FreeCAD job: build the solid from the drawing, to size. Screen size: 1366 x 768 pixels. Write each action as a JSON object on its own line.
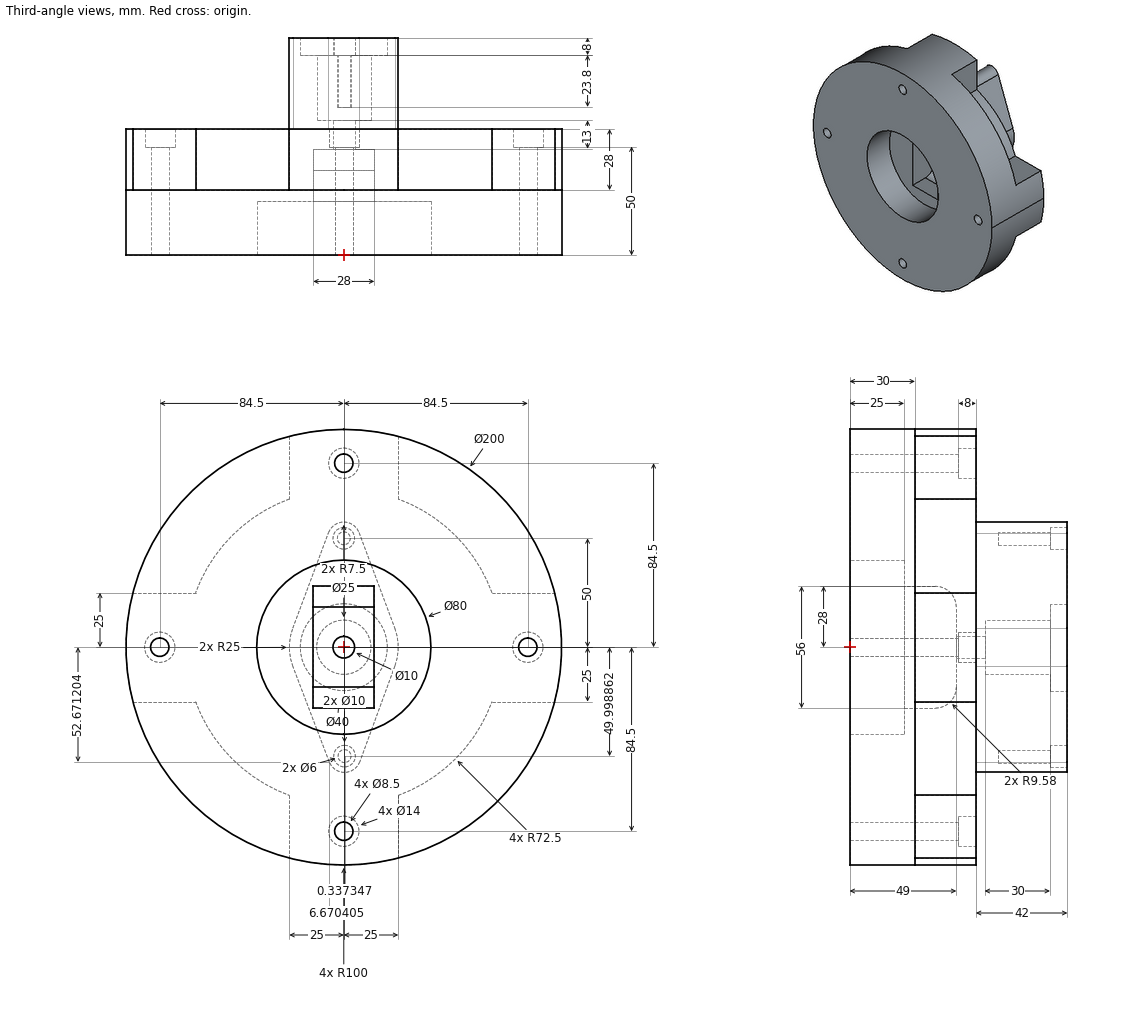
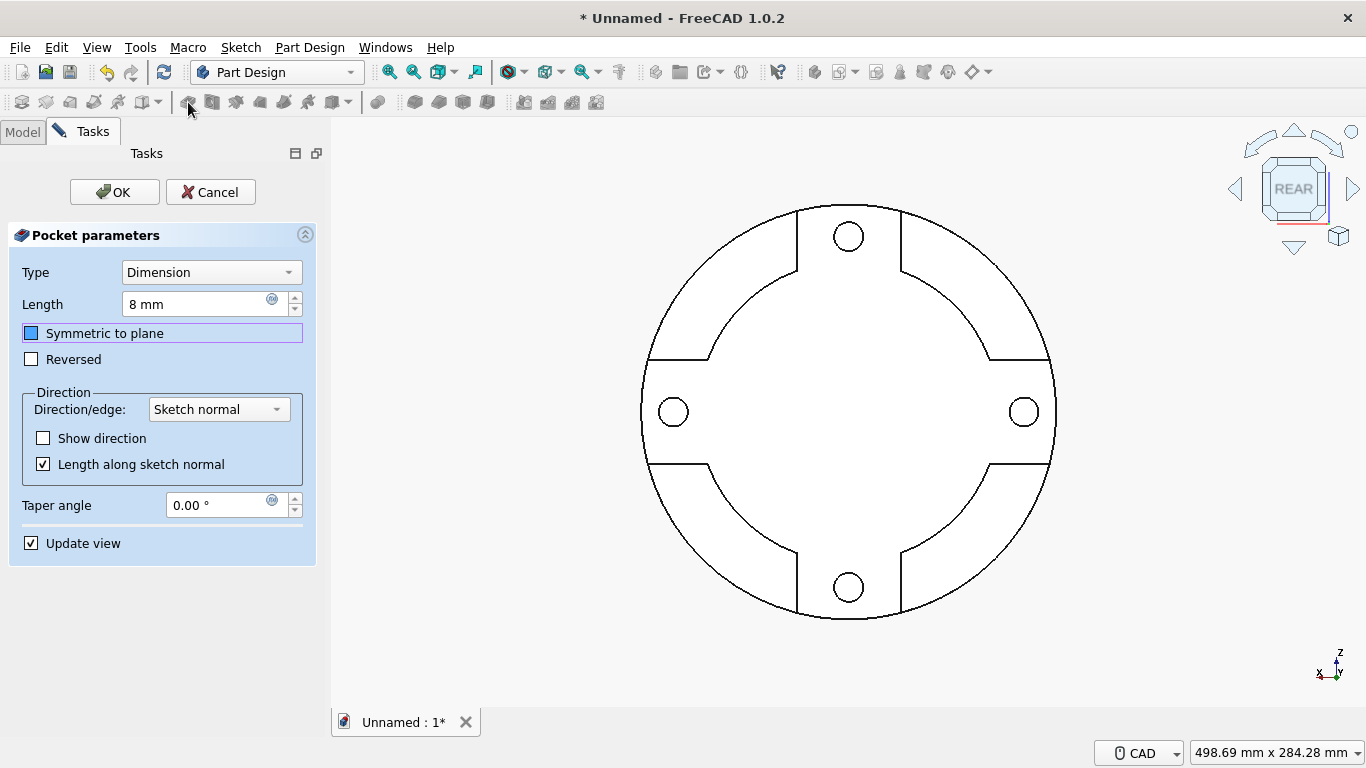
{"action": "left_click", "coordinate": [115, 192]}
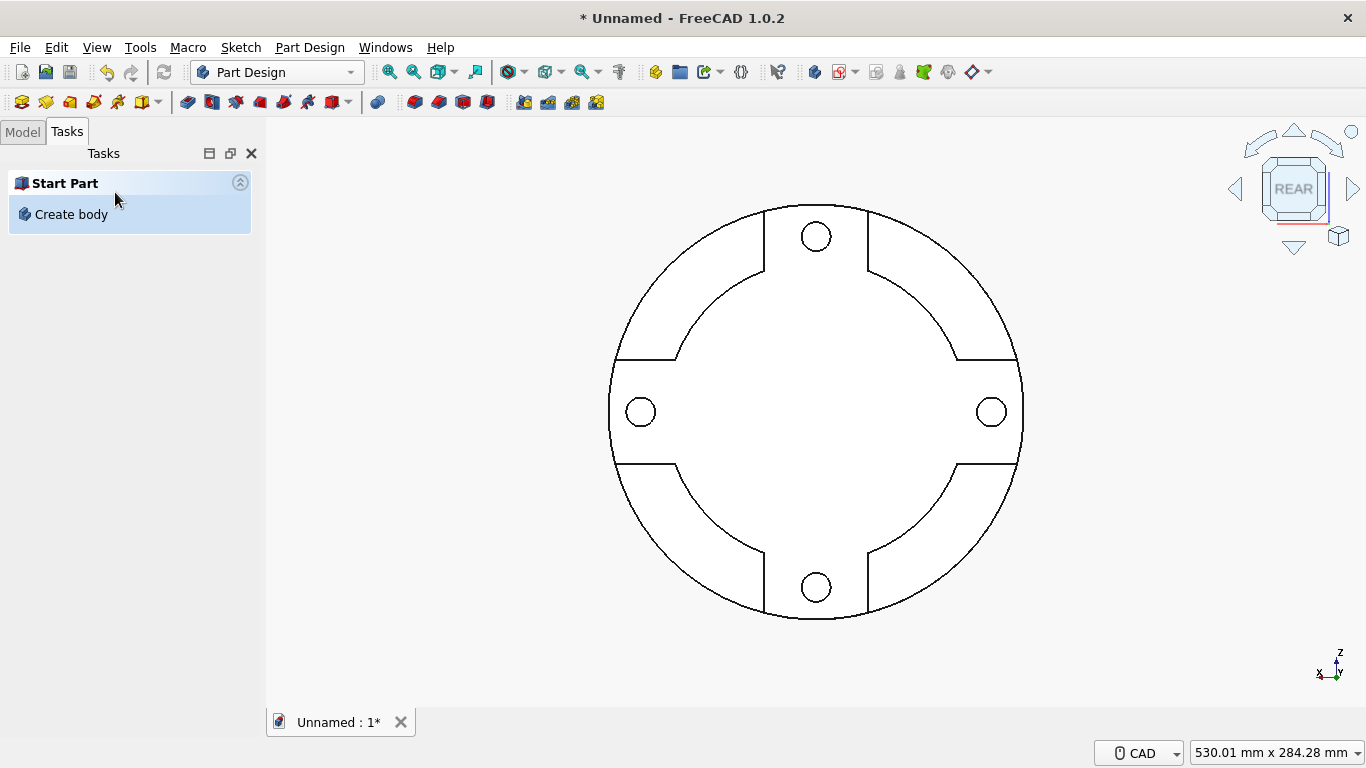
{"action": "left_click", "coordinate": [641, 411]}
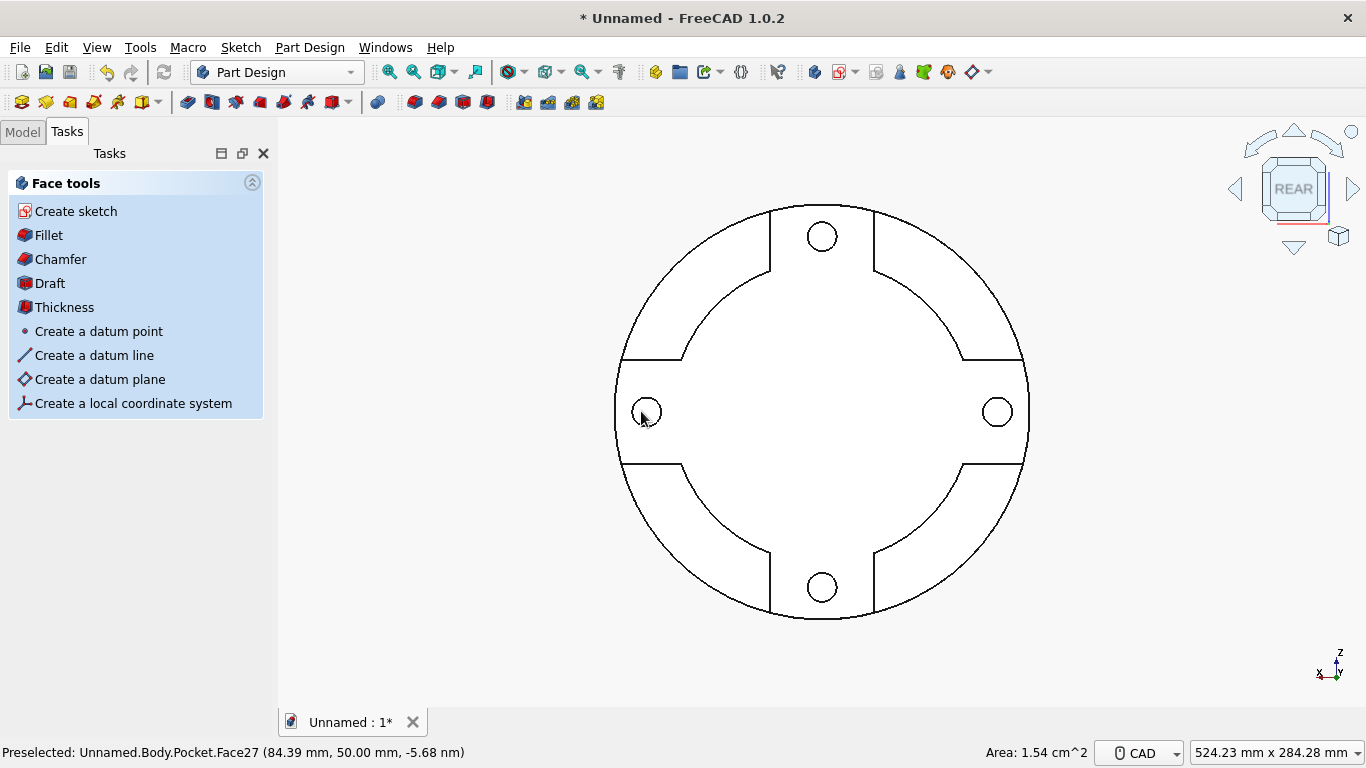
{"action": "left_click", "coordinate": [840, 72]}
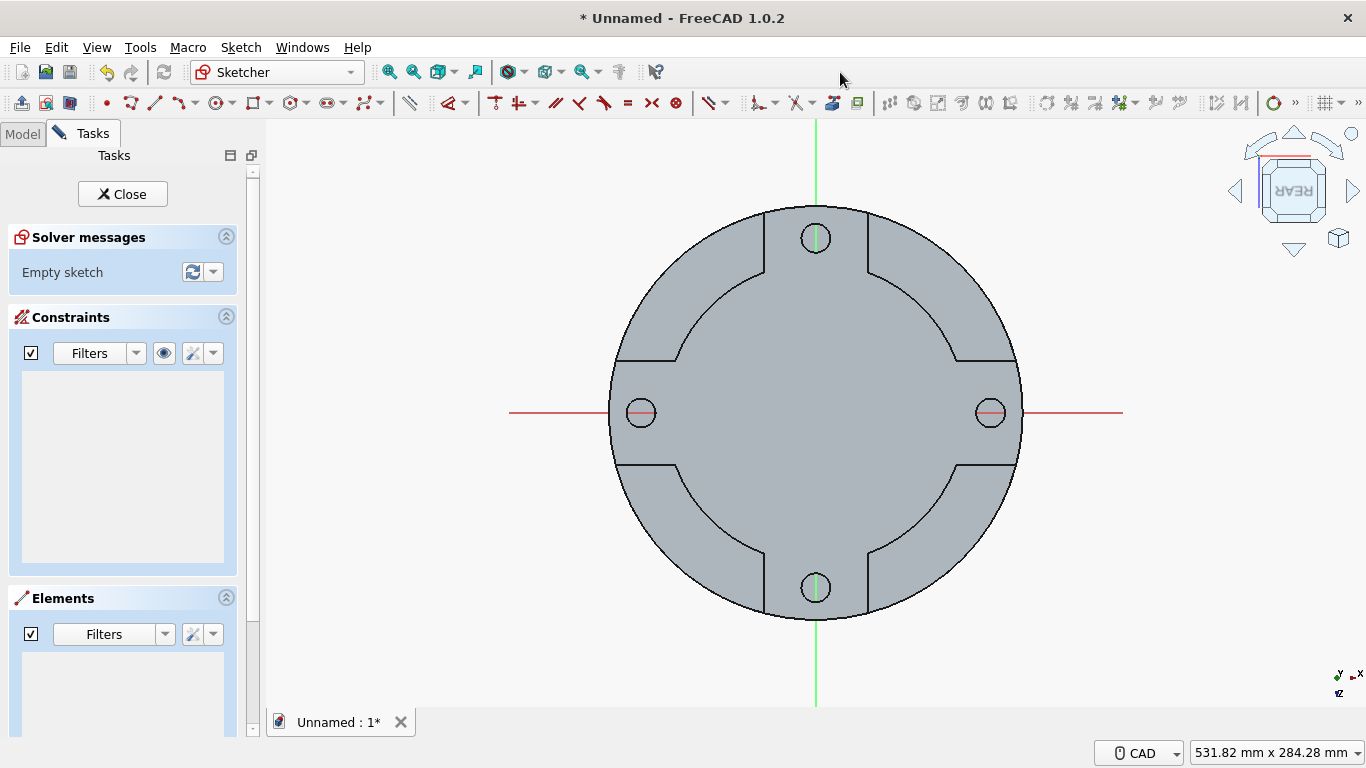
{"action": "key", "text": "g c"}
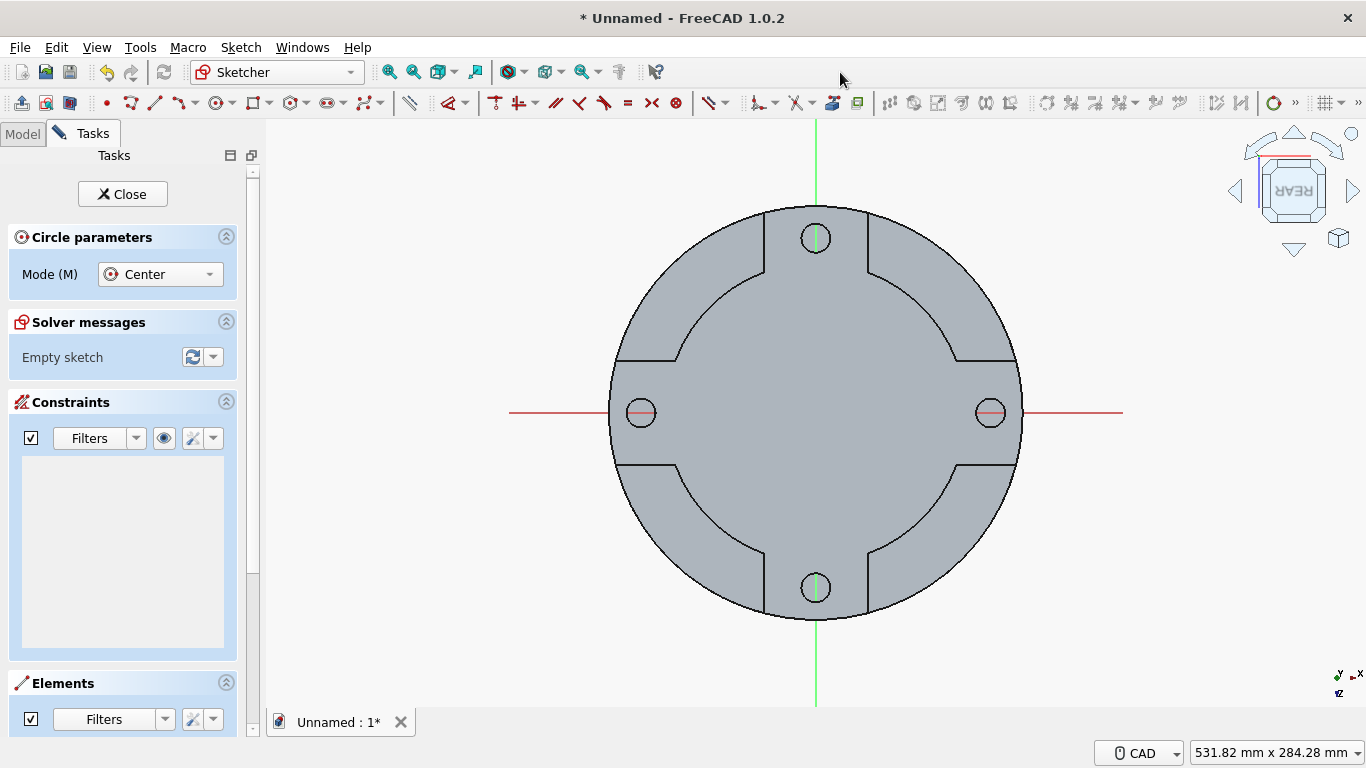
{"action": "scroll", "coordinate": [816, 238], "scroll_direction": "up", "scroll_amount": 5}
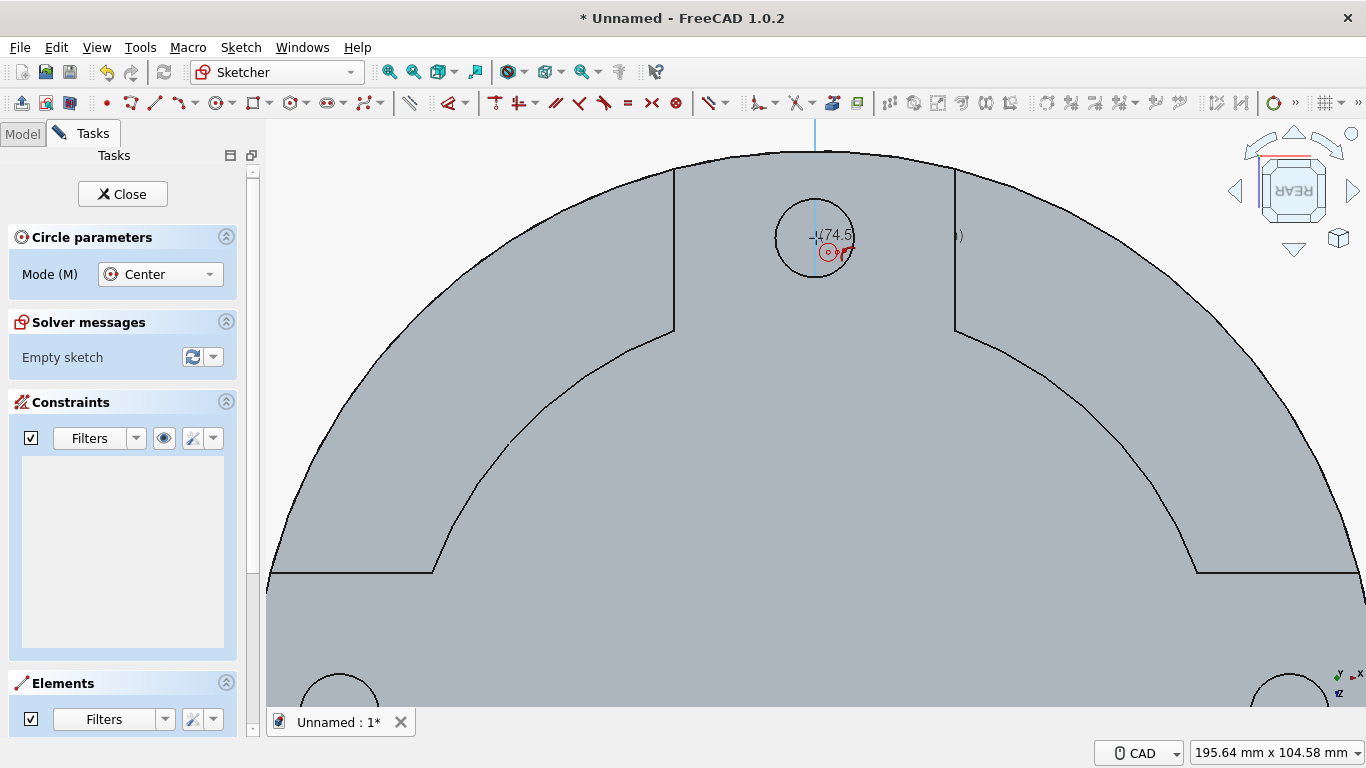
{"action": "left_click", "coordinate": [815, 238]}
{"action": "left_click", "coordinate": [832, 221]}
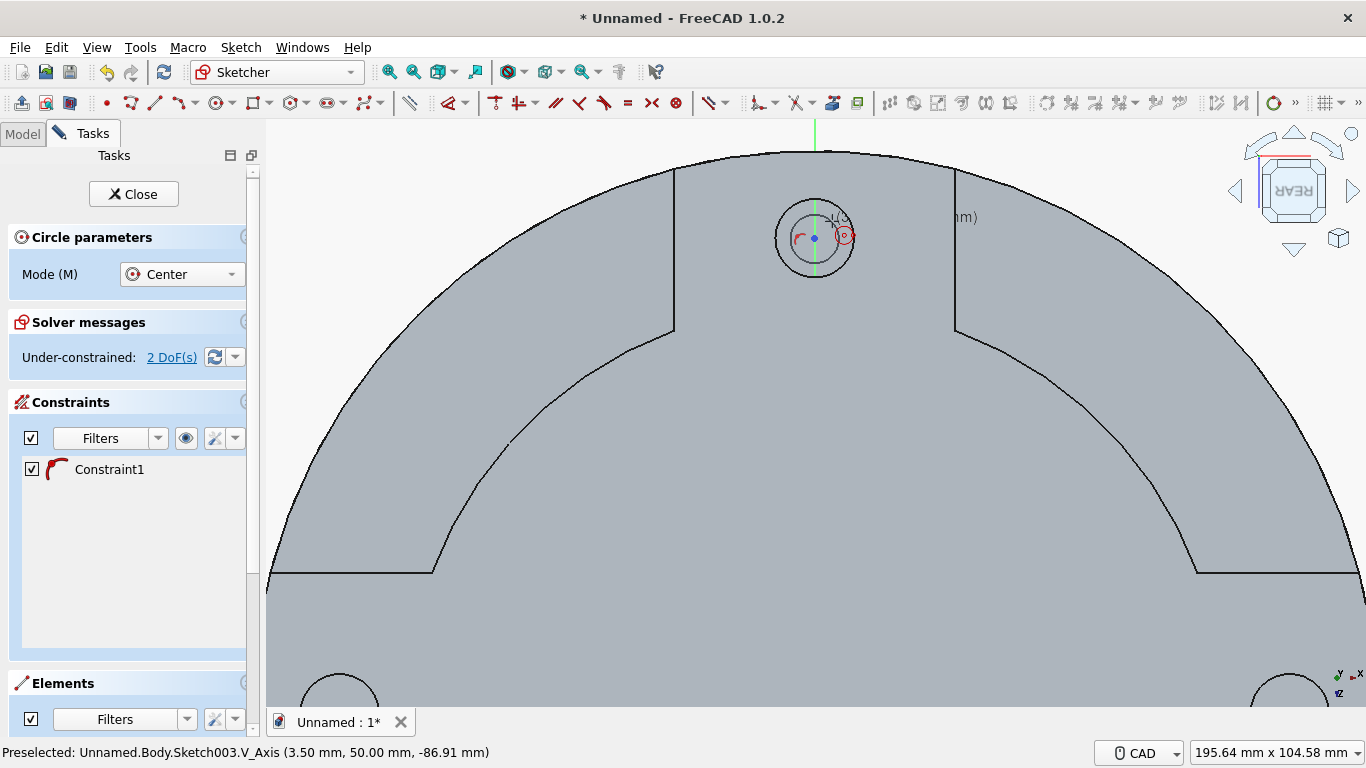
{"action": "scroll", "coordinate": [708, 238], "scroll_direction": "down", "scroll_amount": 5}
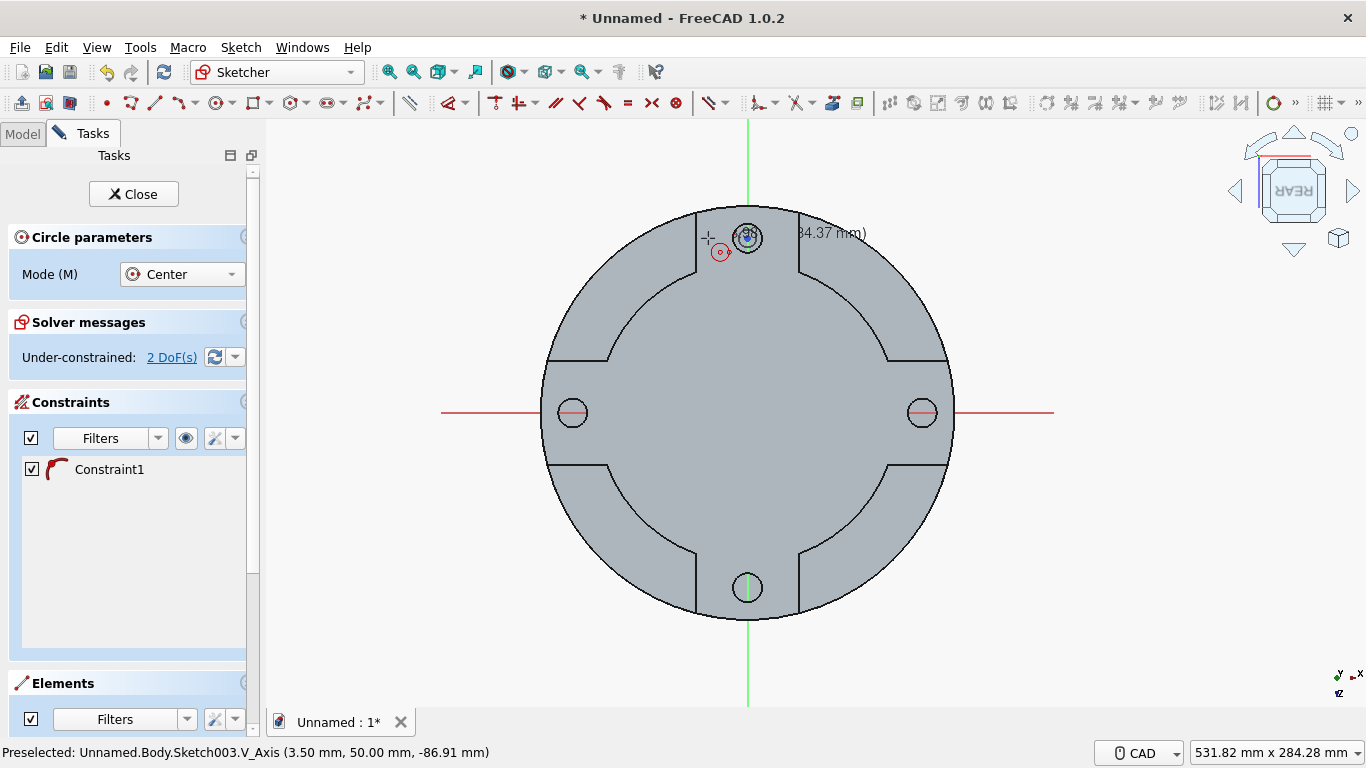
{"action": "scroll", "coordinate": [922, 413], "scroll_direction": "up", "scroll_amount": 5}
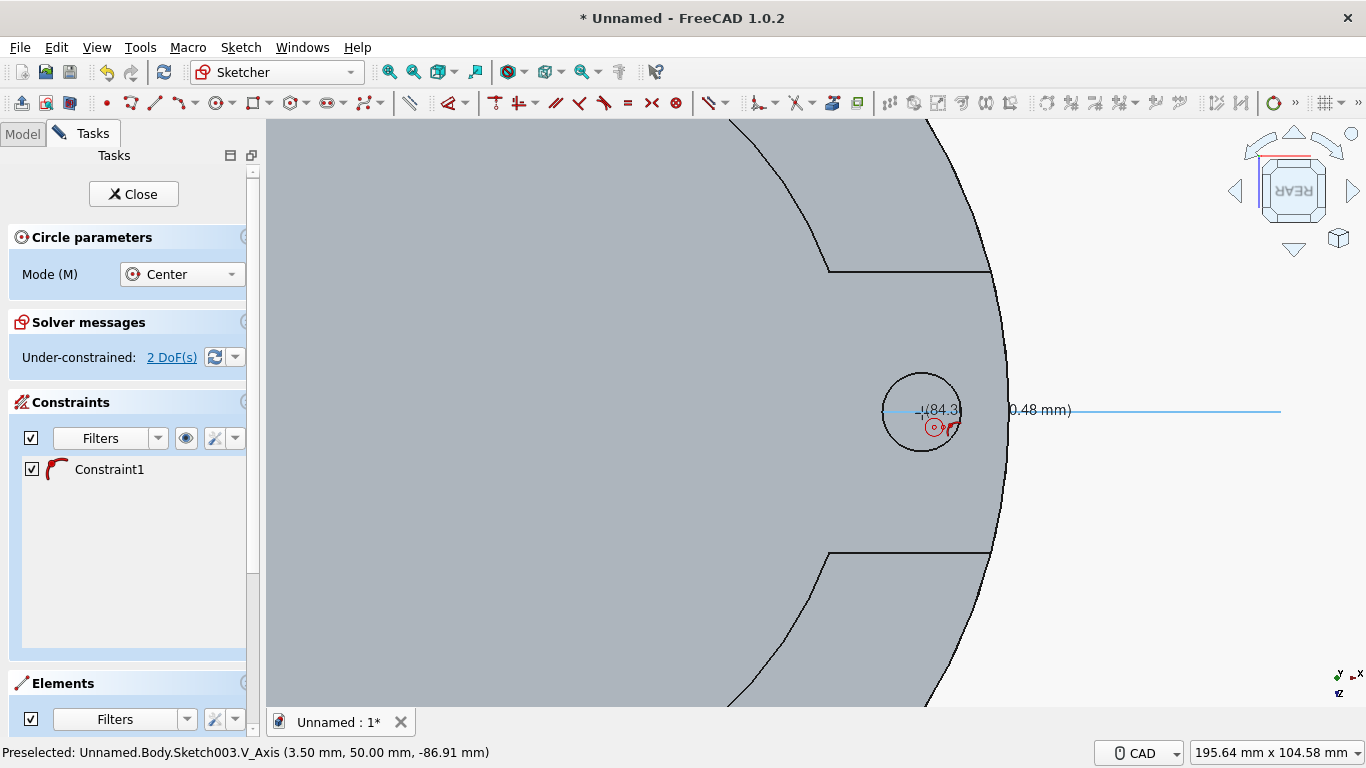
{"action": "left_click", "coordinate": [922, 412]}
{"action": "left_click", "coordinate": [939, 395]}